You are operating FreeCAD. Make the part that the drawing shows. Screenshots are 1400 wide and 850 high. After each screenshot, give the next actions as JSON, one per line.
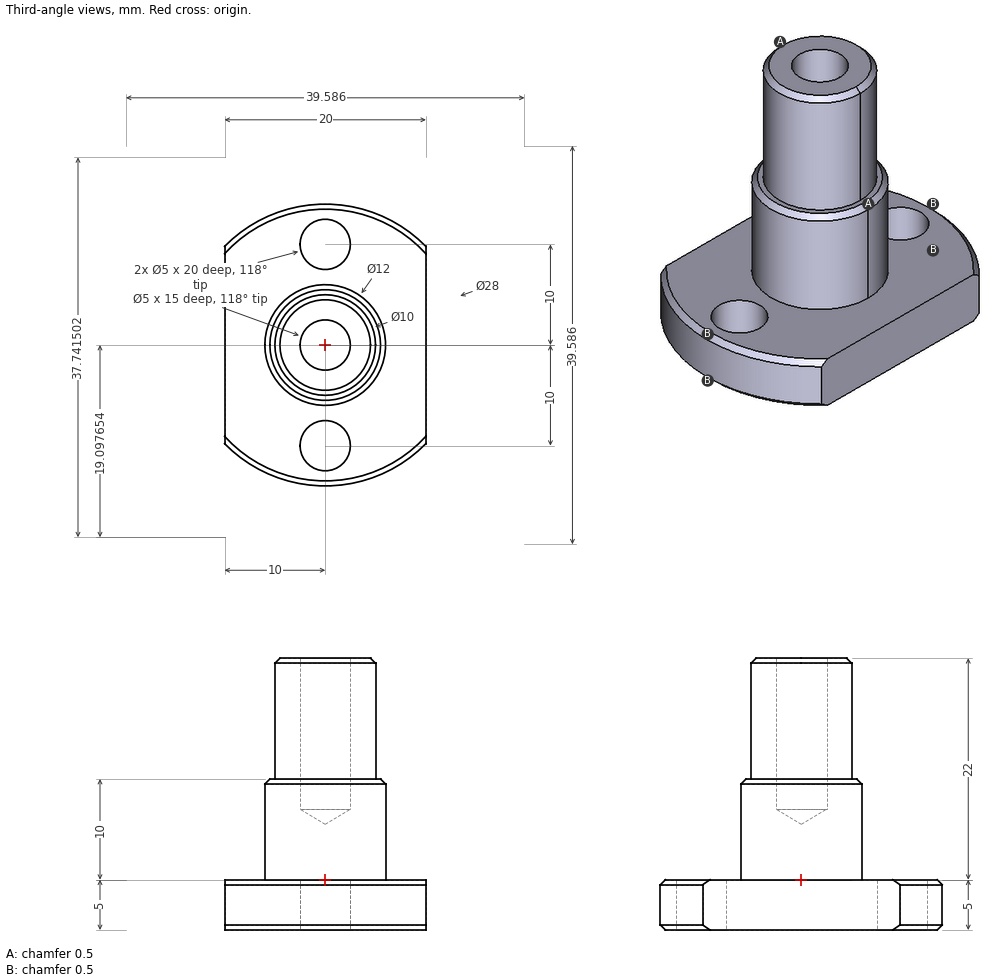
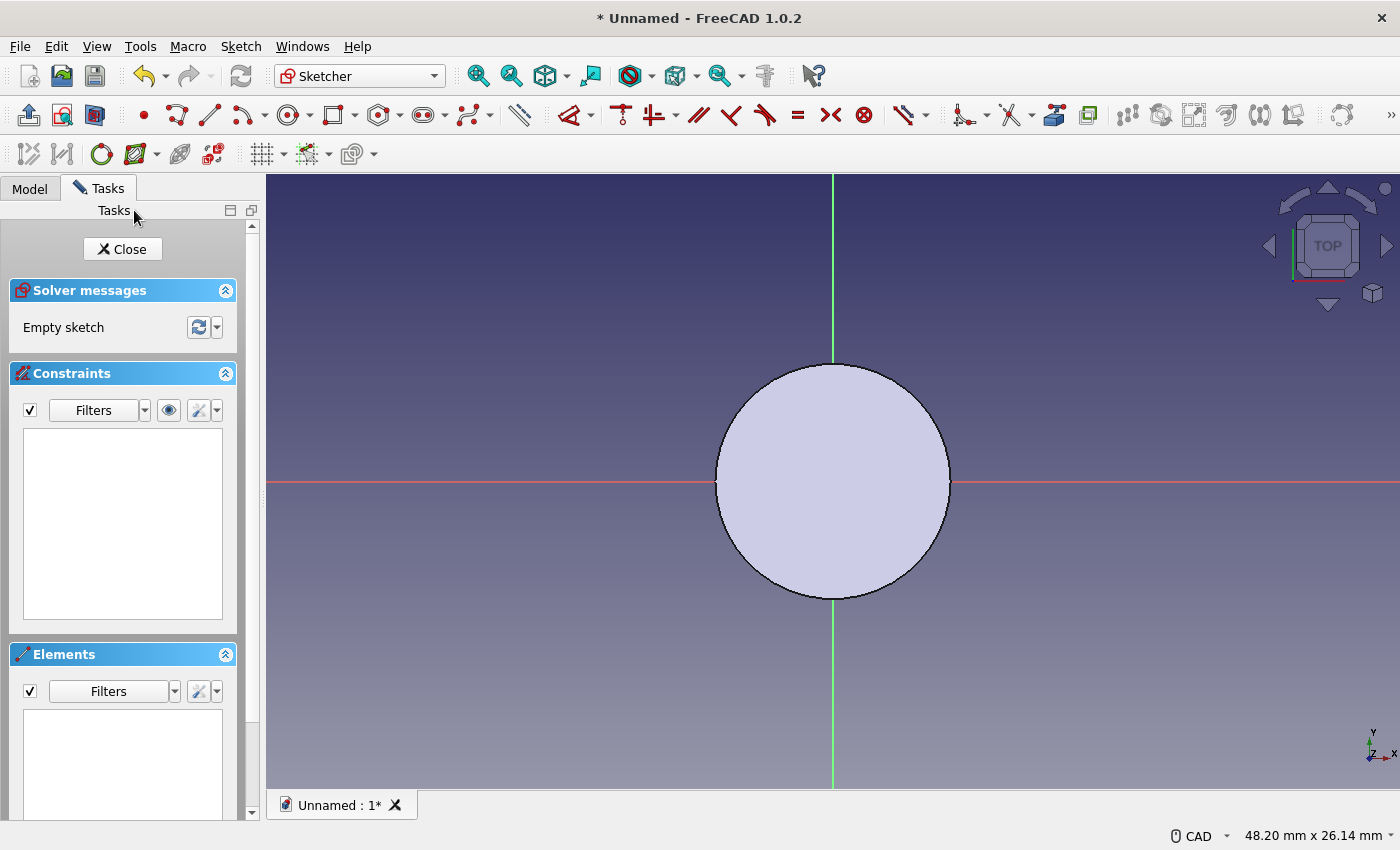
{"action": "key", "text": "q s"}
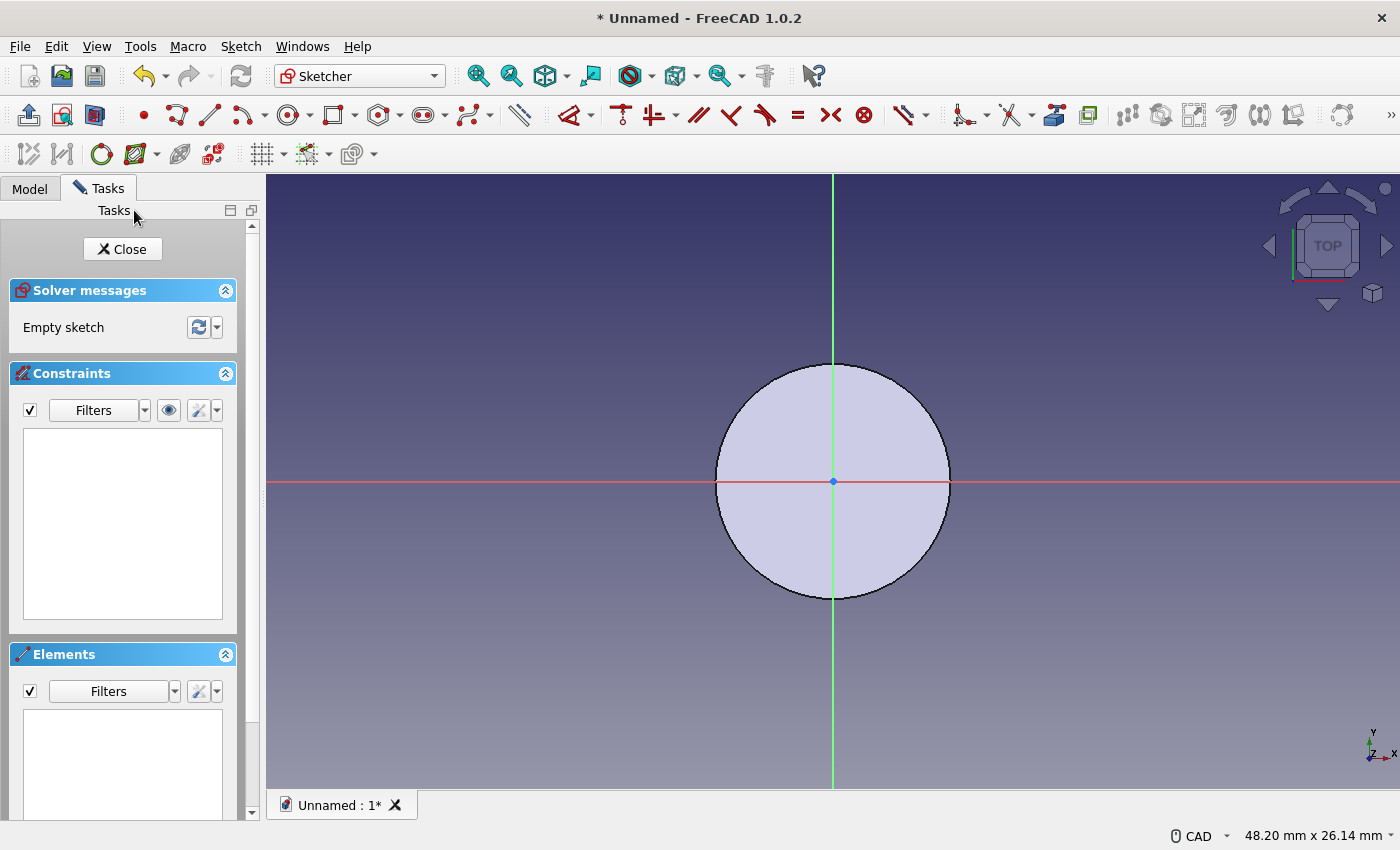
{"action": "scroll", "coordinate": [972, 482], "scroll_direction": "up", "scroll_amount": 2}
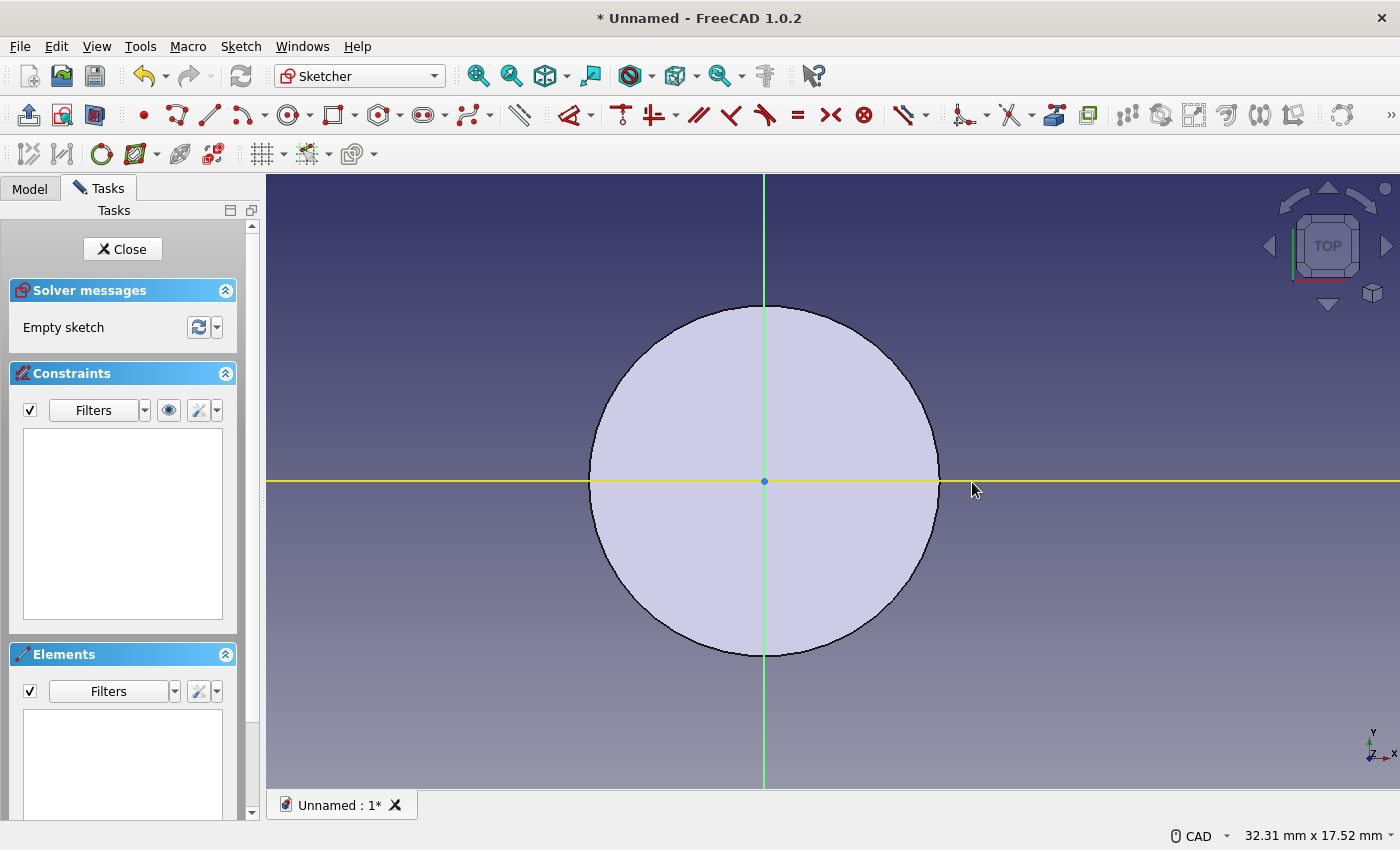
{"action": "left_click", "coordinate": [288, 116]}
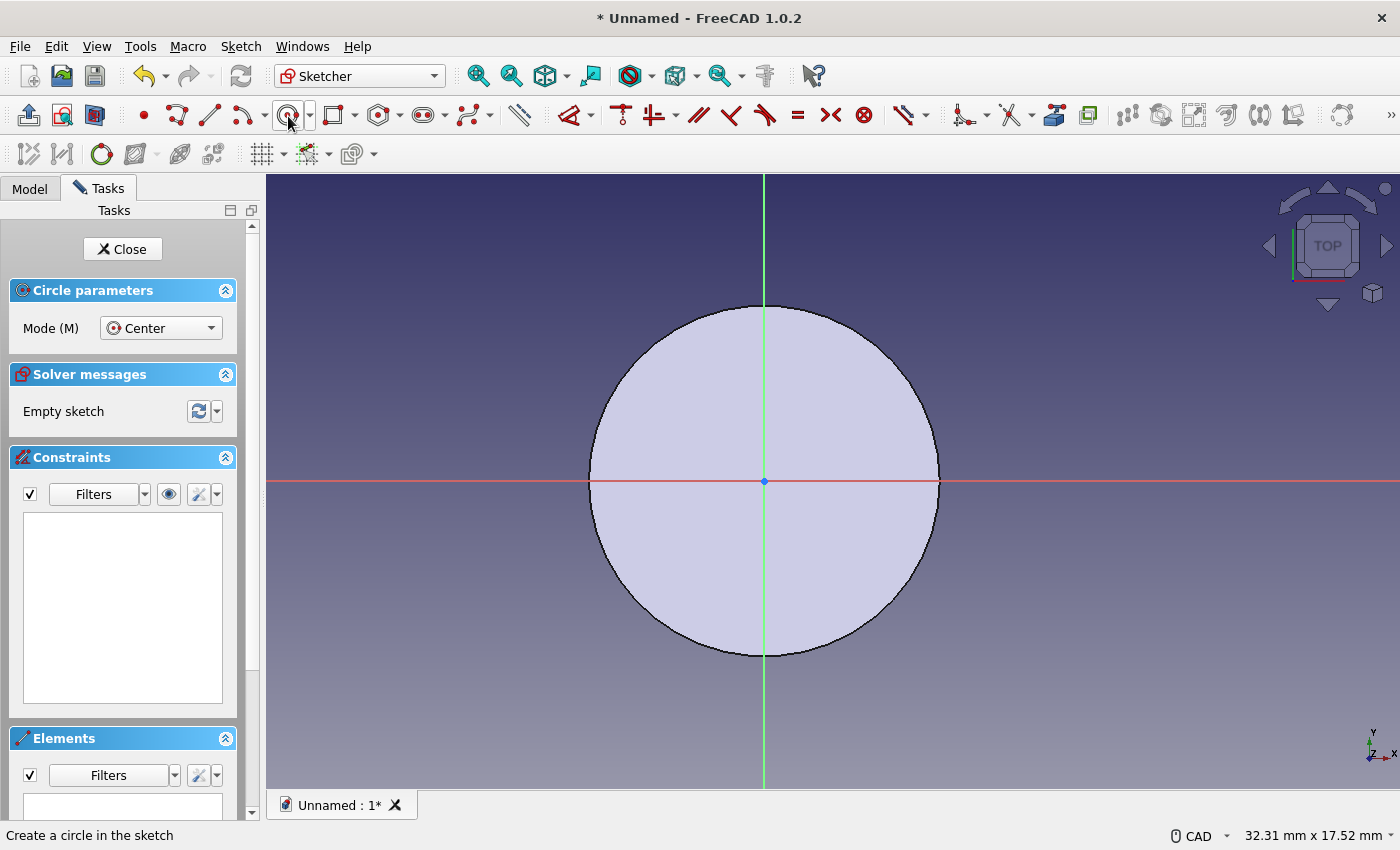
{"action": "left_click", "coordinate": [764, 481]}
{"action": "mouse_move", "coordinate": [913, 332]}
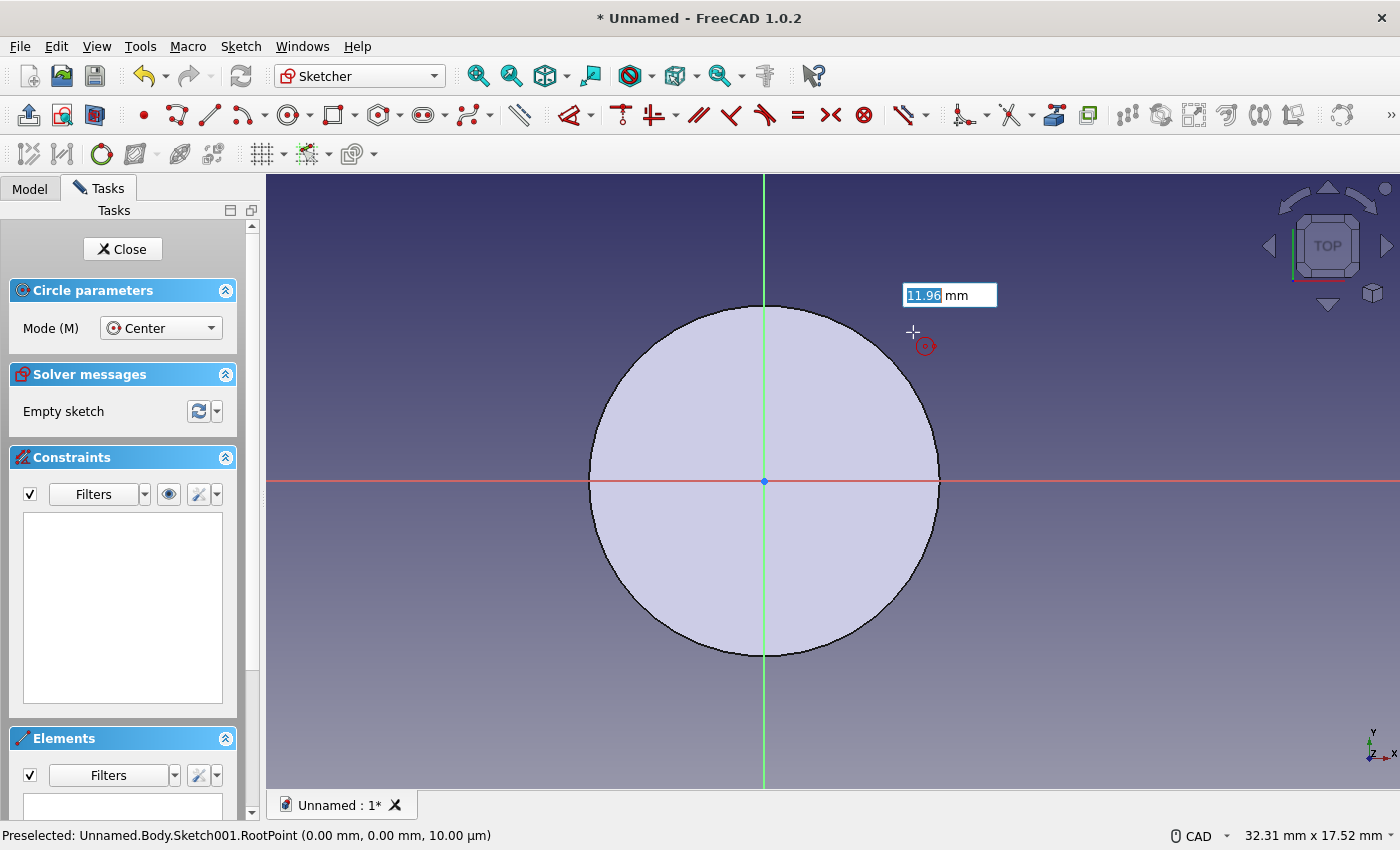
{"action": "type", "text": "12"}
{"action": "key", "text": "Return"}
{"action": "key", "text": "Escape"}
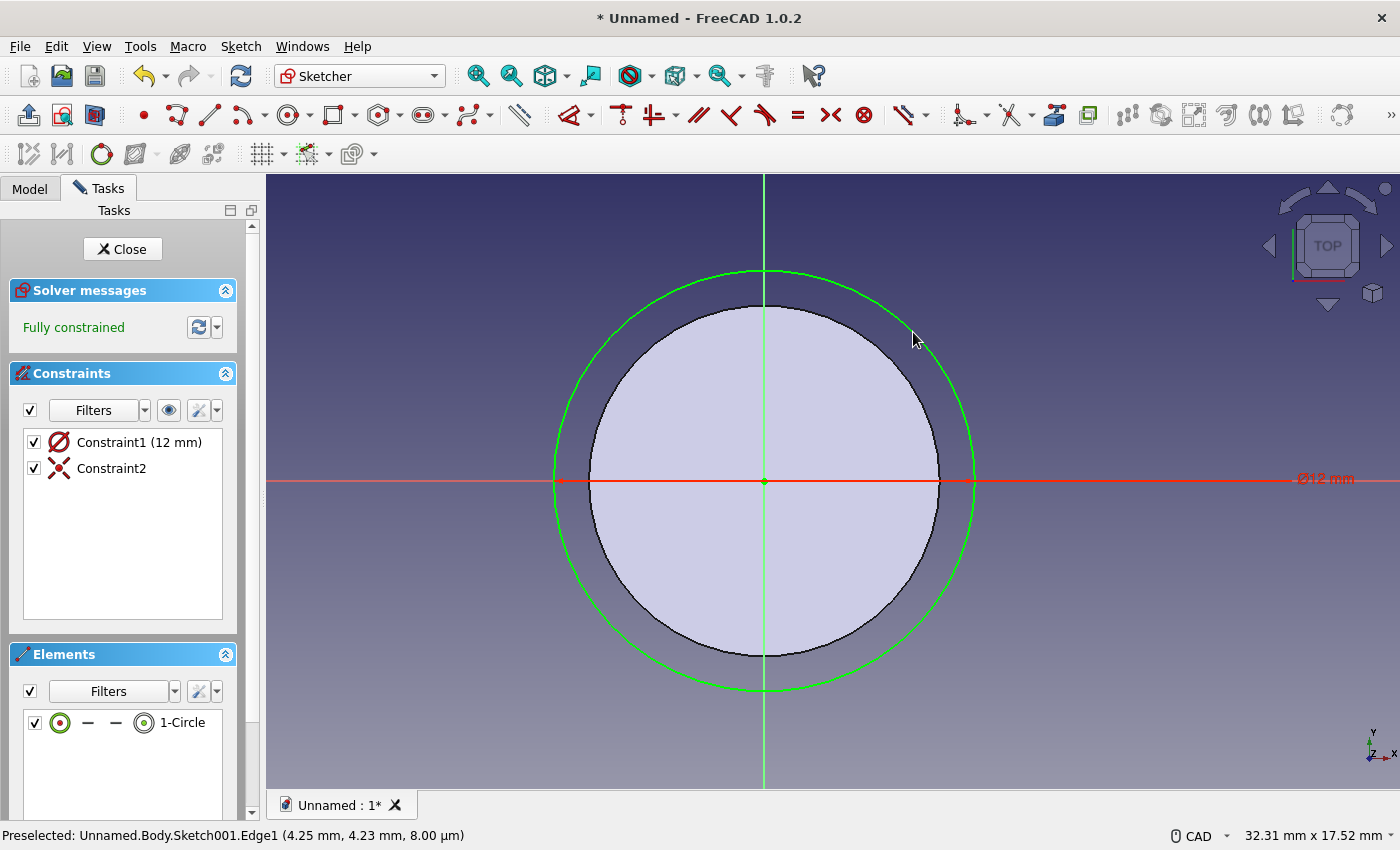
{"action": "left_click", "coordinate": [123, 249]}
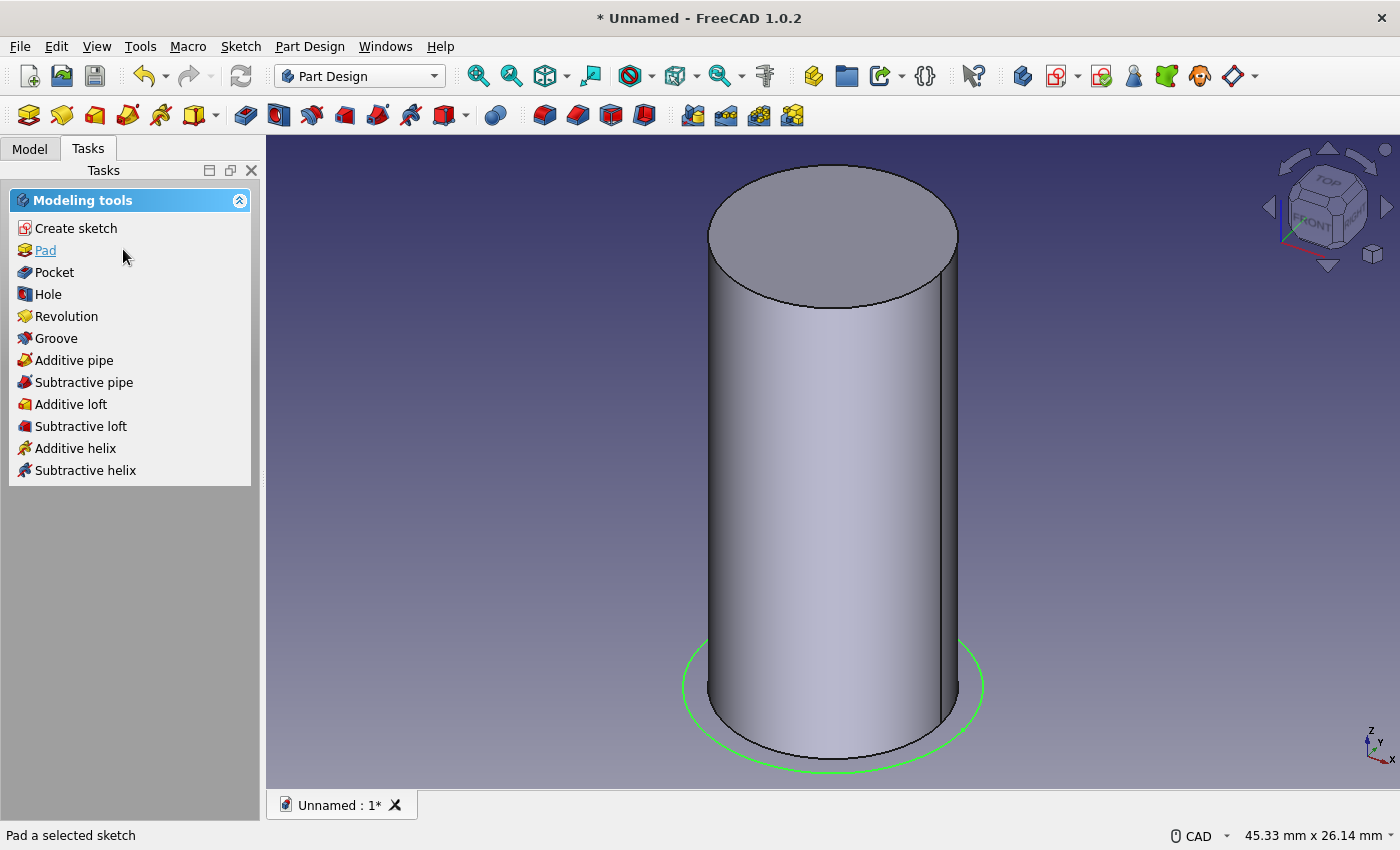
{"action": "left_click", "coordinate": [29, 116]}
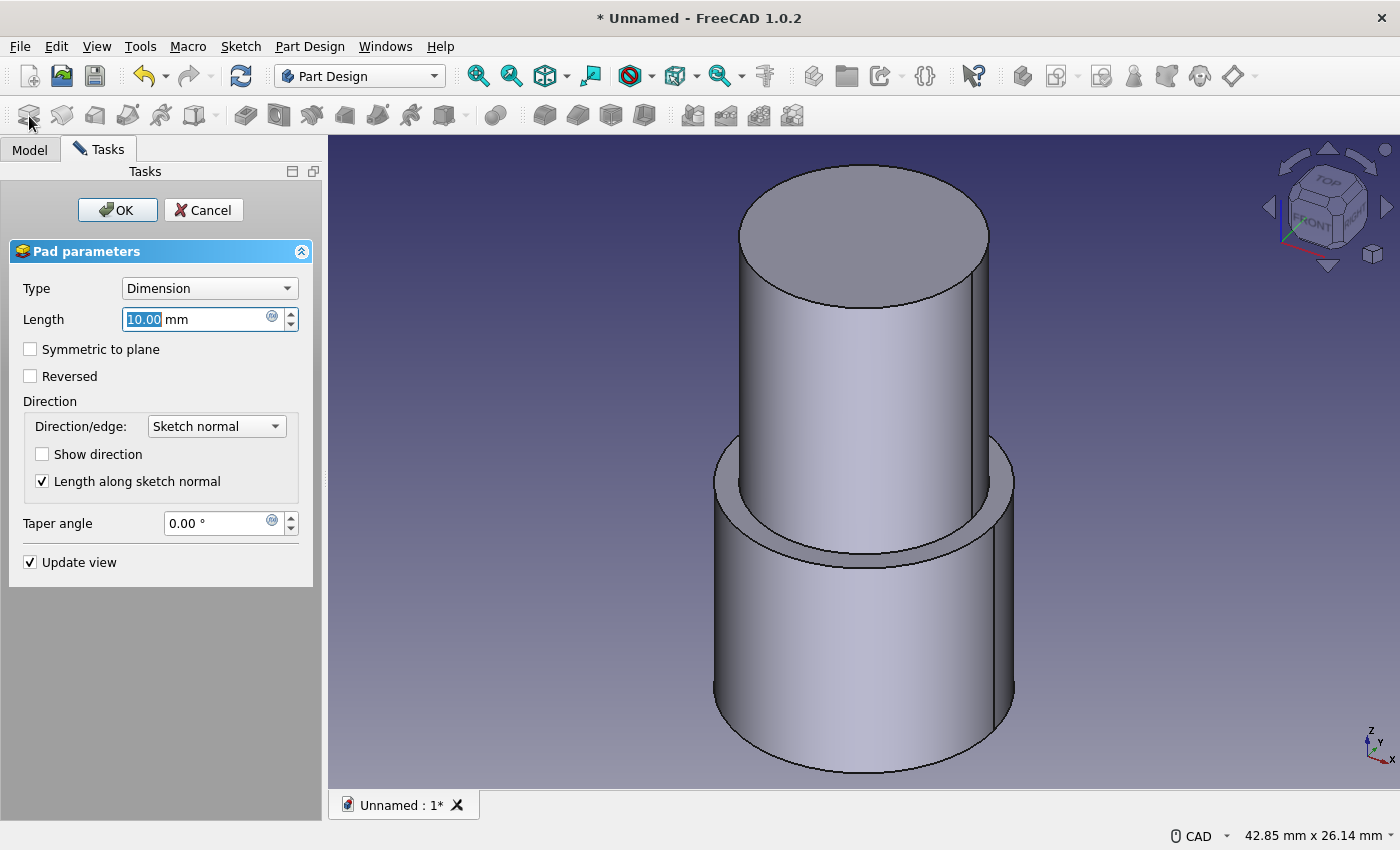
{"action": "type", "text": "10"}
{"action": "key", "text": "Tab"}